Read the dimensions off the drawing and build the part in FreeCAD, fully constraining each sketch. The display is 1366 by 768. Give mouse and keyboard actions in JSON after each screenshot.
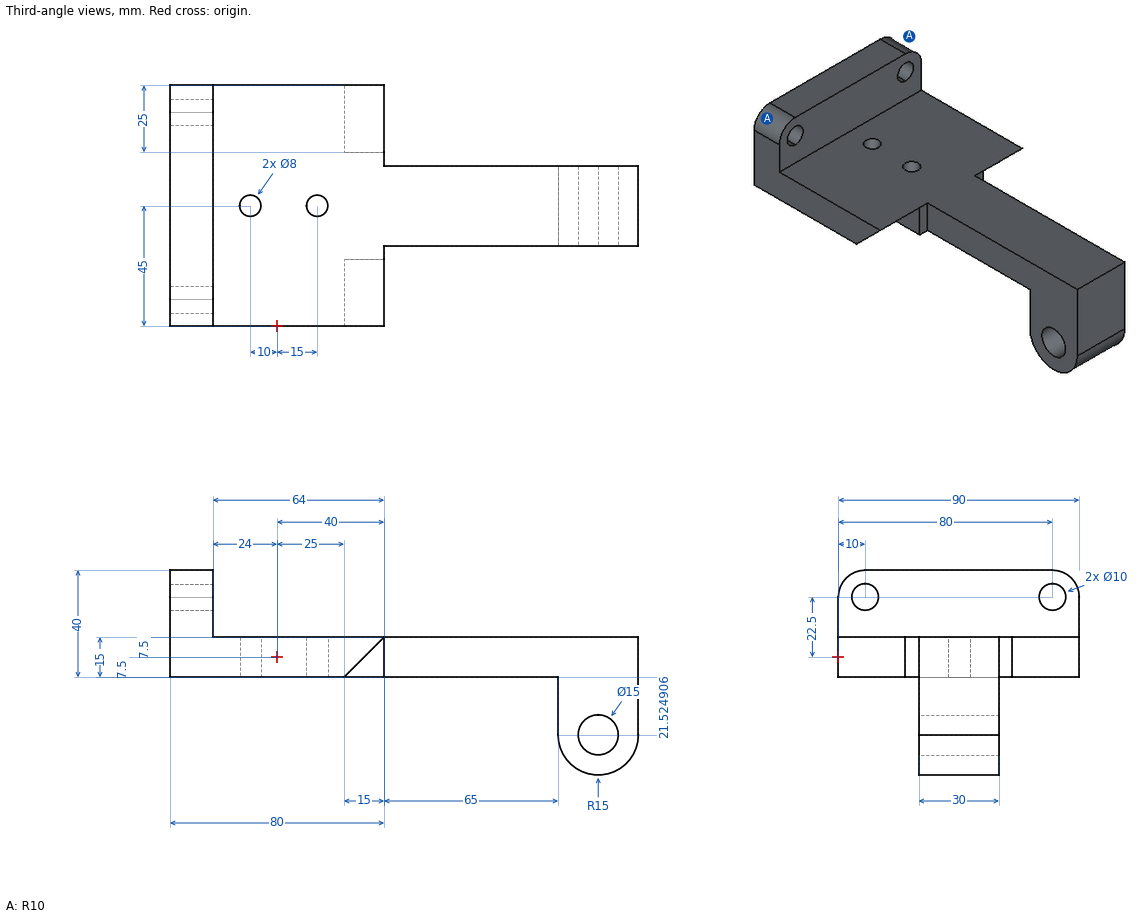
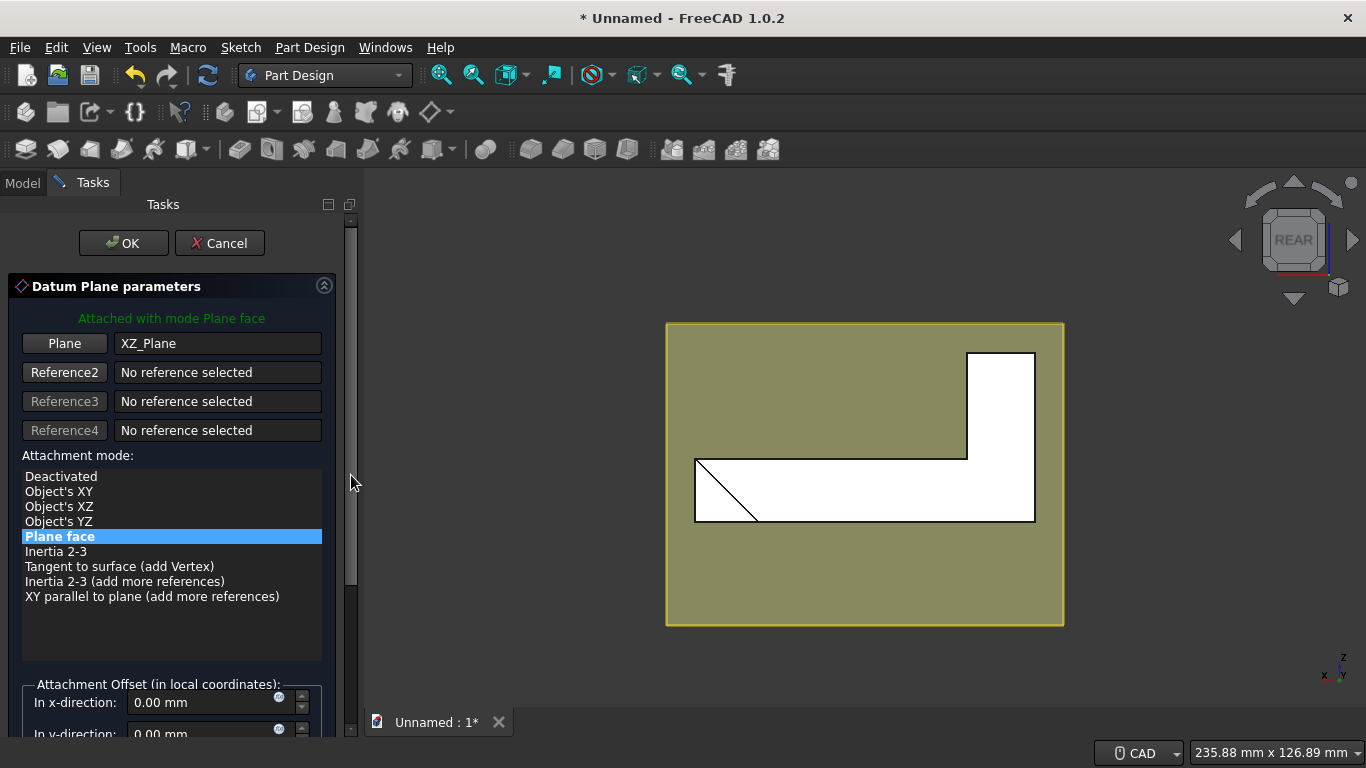
{"action": "left_click", "coordinate": [124, 243]}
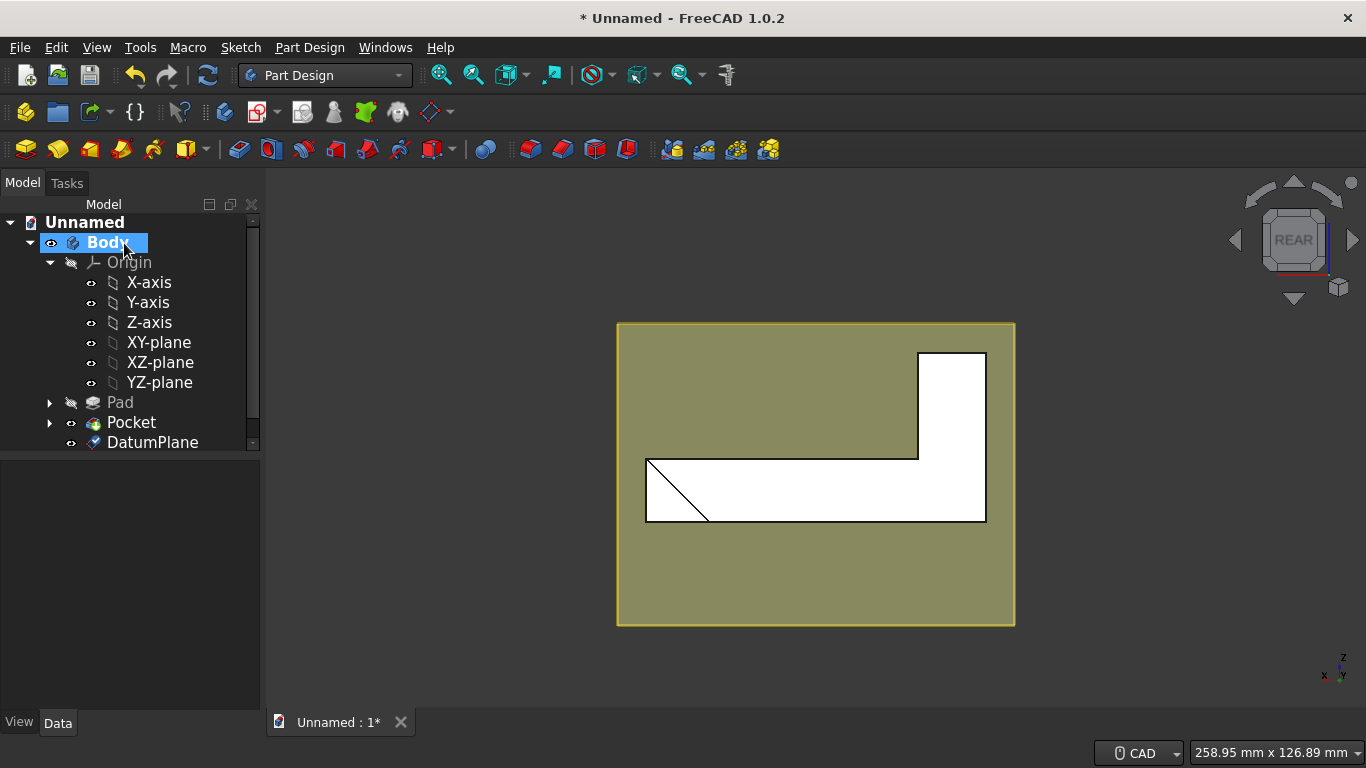
{"action": "left_click", "coordinate": [116, 423]}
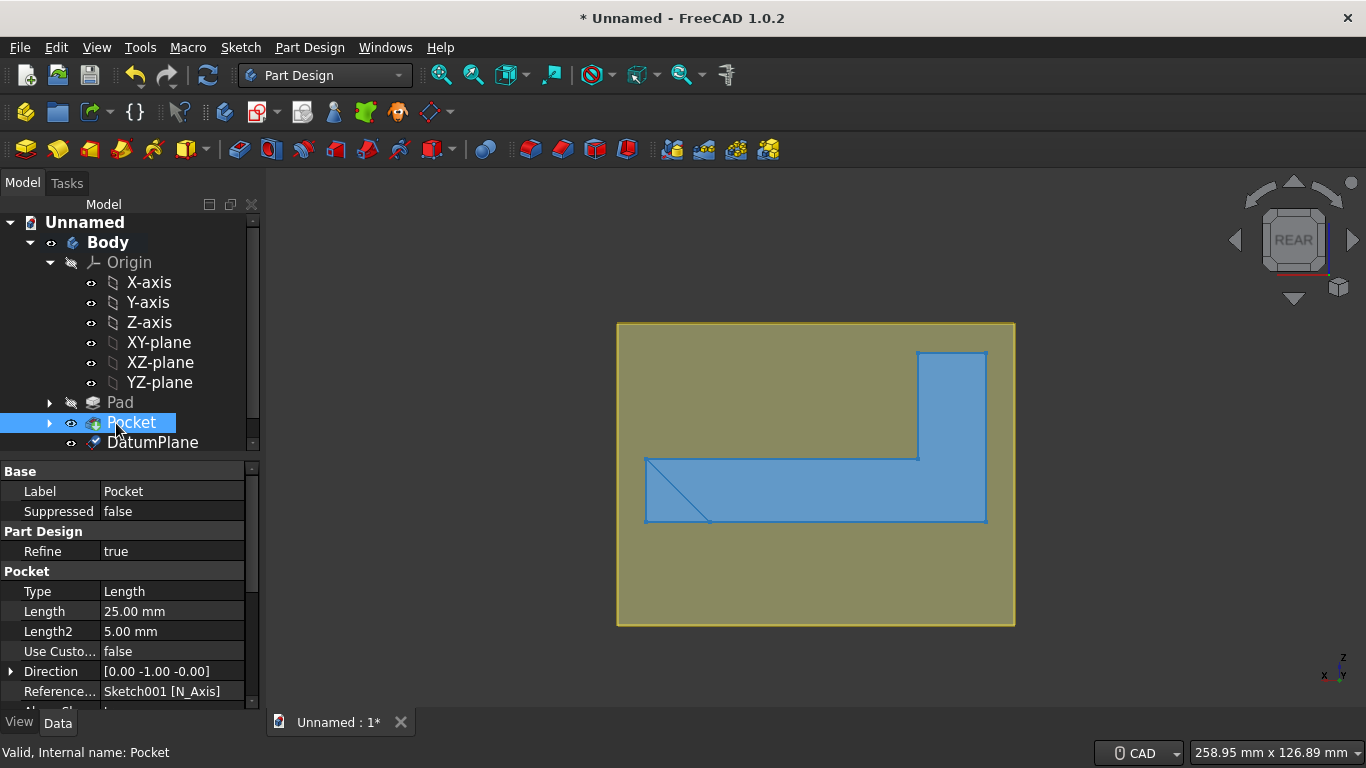
{"action": "left_click", "coordinate": [672, 150]}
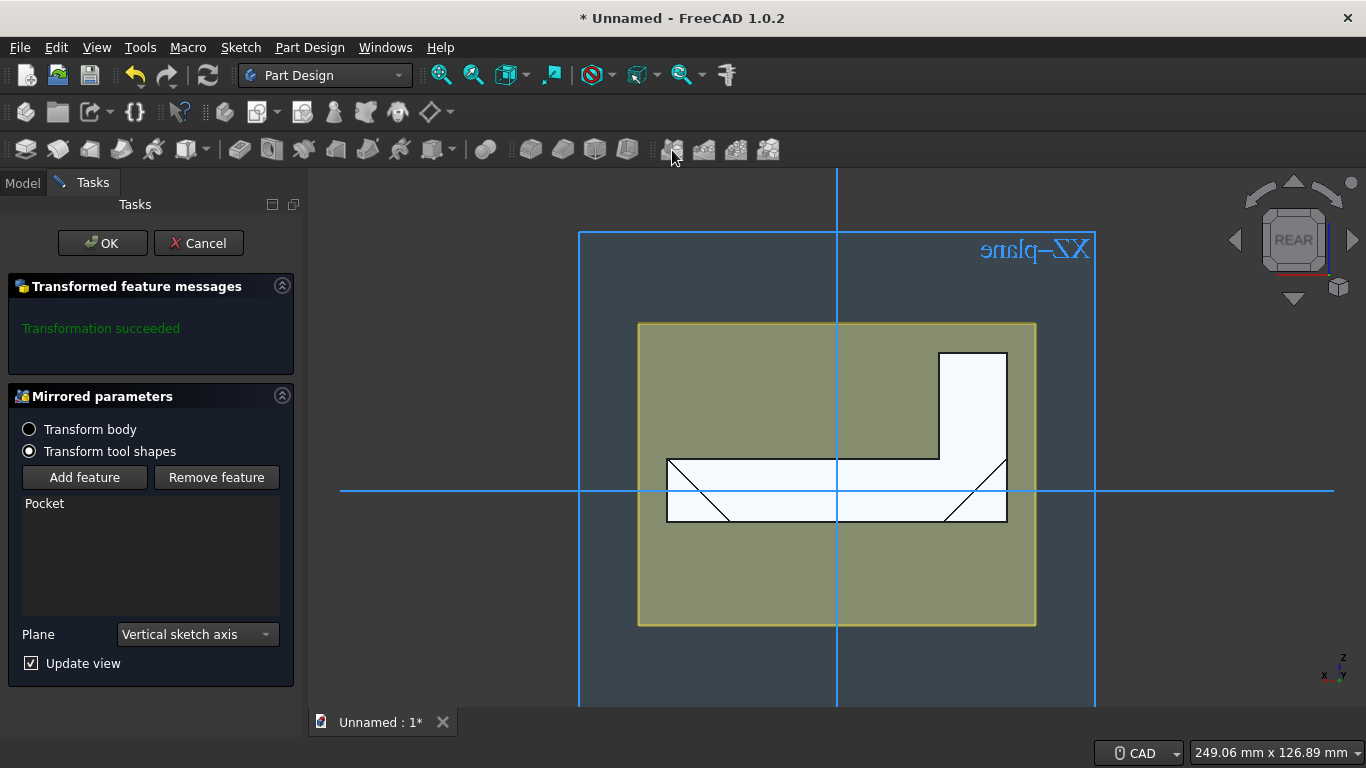
{"action": "left_click", "coordinate": [198, 634]}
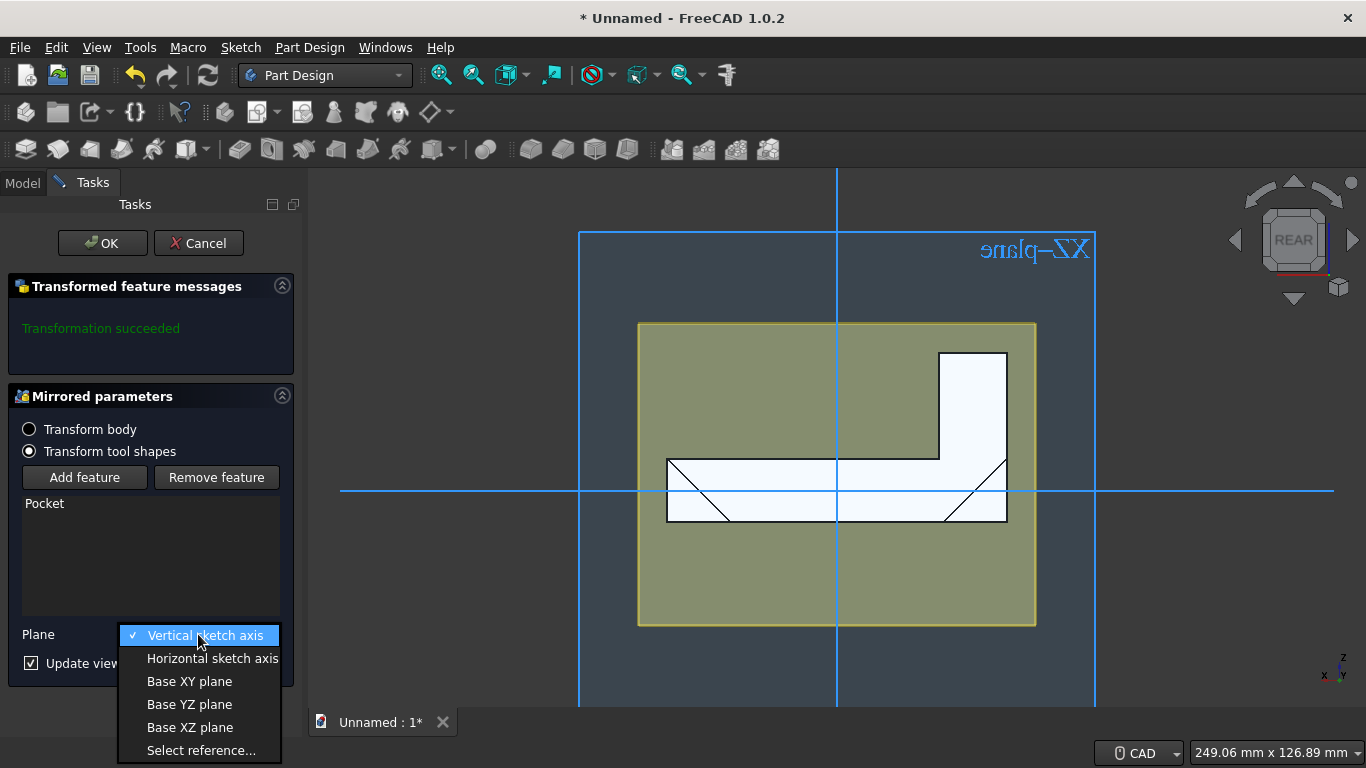
{"action": "left_click", "coordinate": [198, 750]}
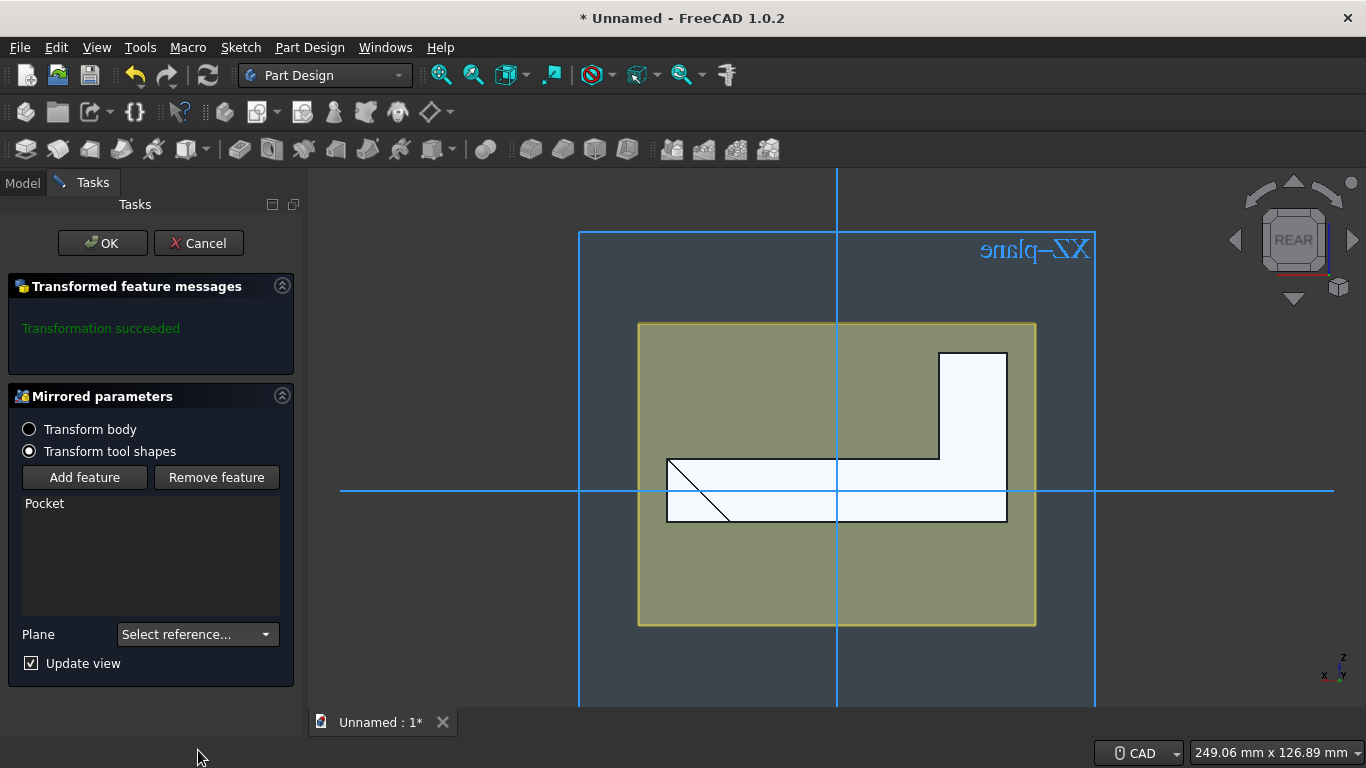
{"action": "left_click", "coordinate": [23, 182]}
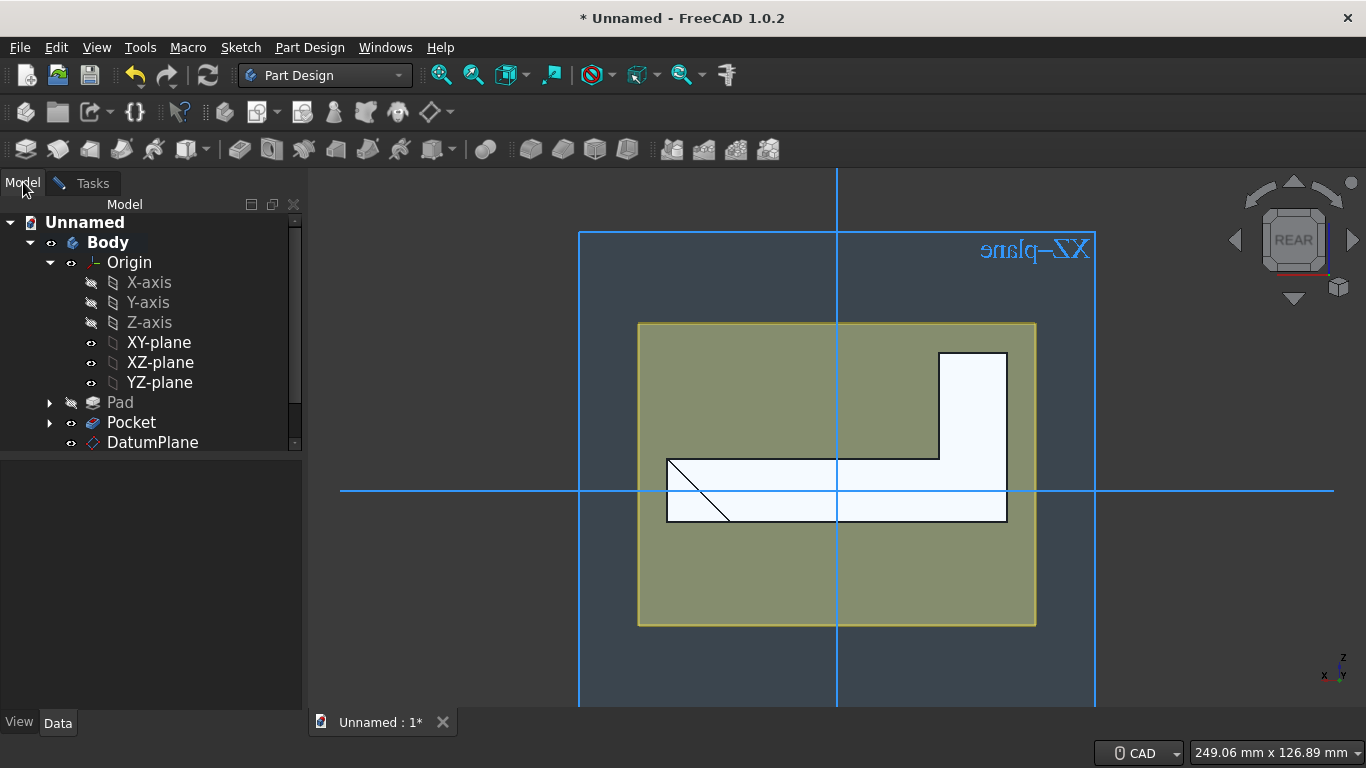
{"action": "left_click", "coordinate": [116, 443]}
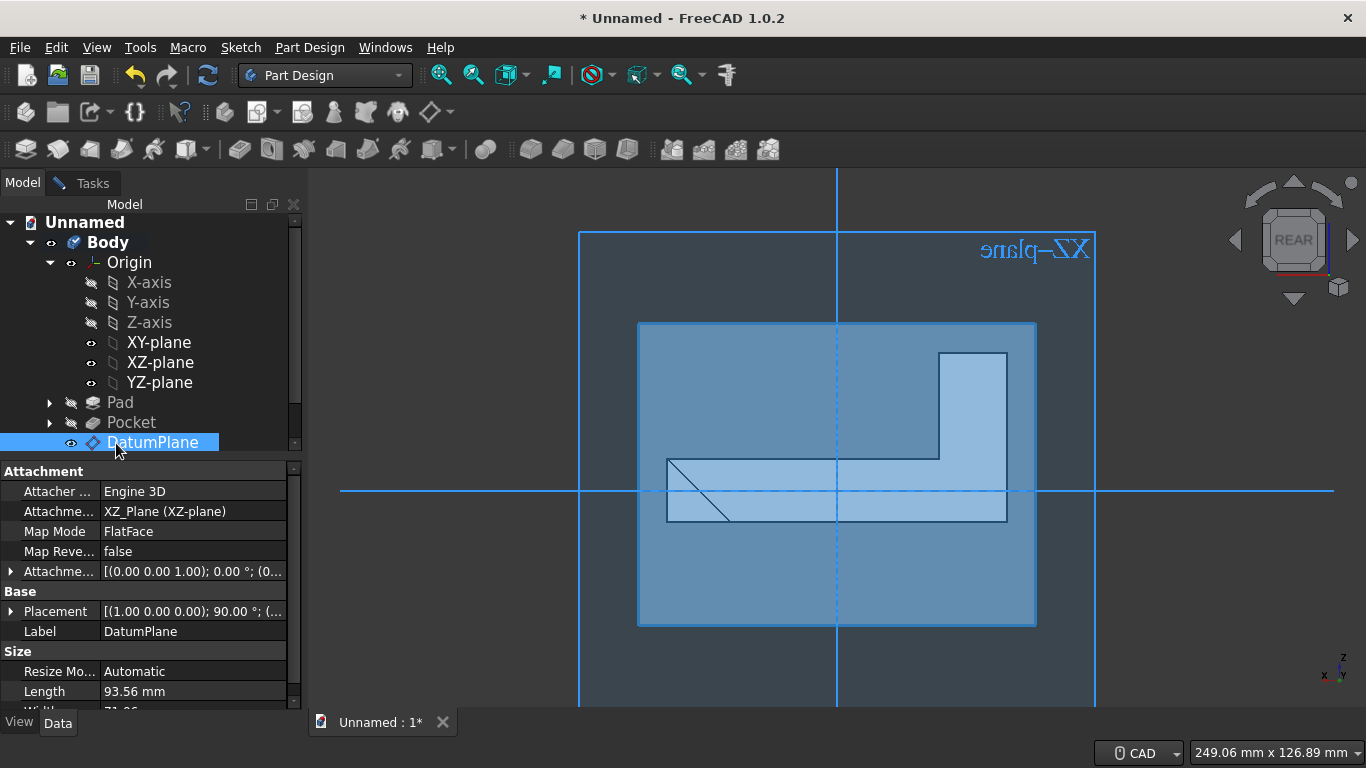
{"action": "left_click", "coordinate": [84, 182]}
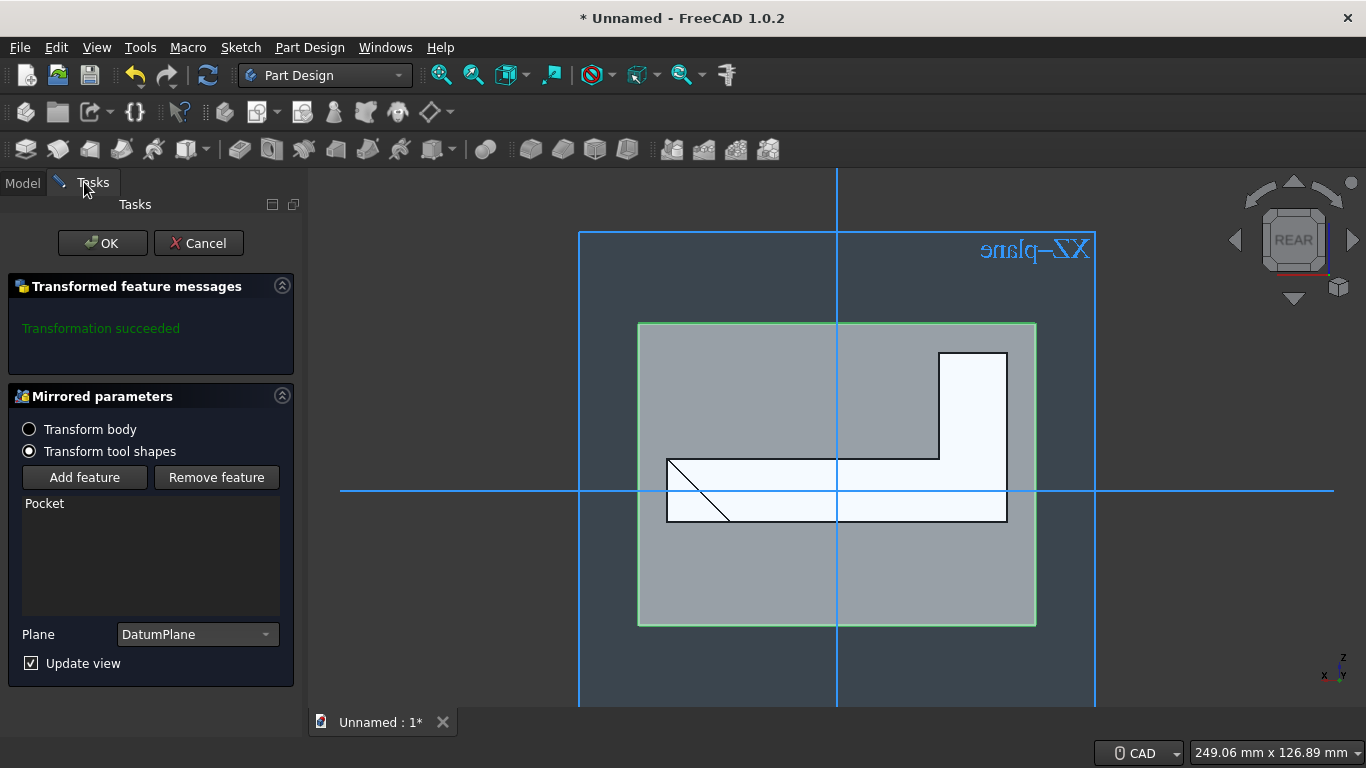
{"action": "left_click", "coordinate": [103, 243]}